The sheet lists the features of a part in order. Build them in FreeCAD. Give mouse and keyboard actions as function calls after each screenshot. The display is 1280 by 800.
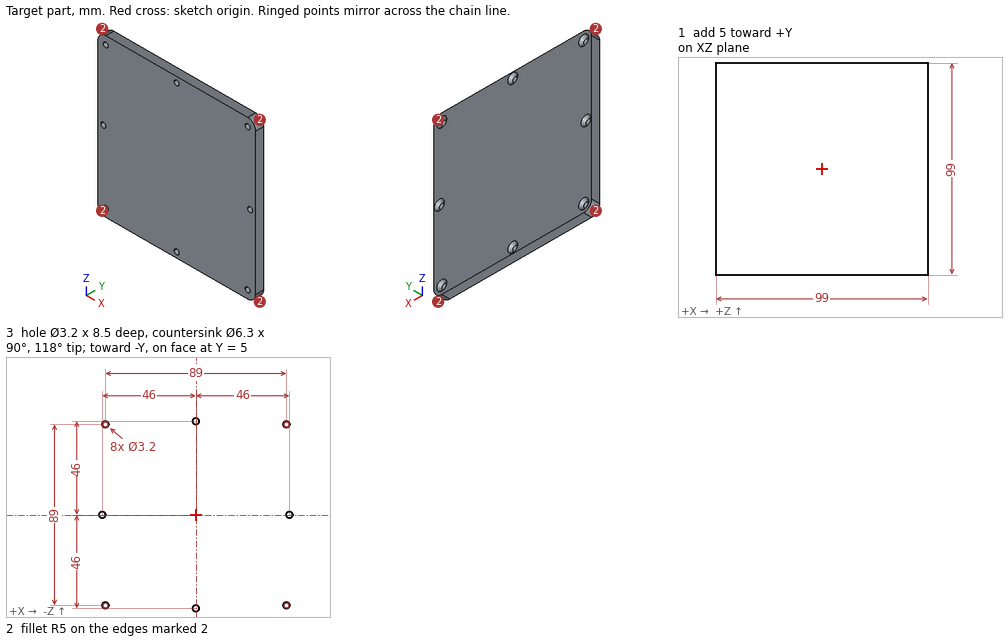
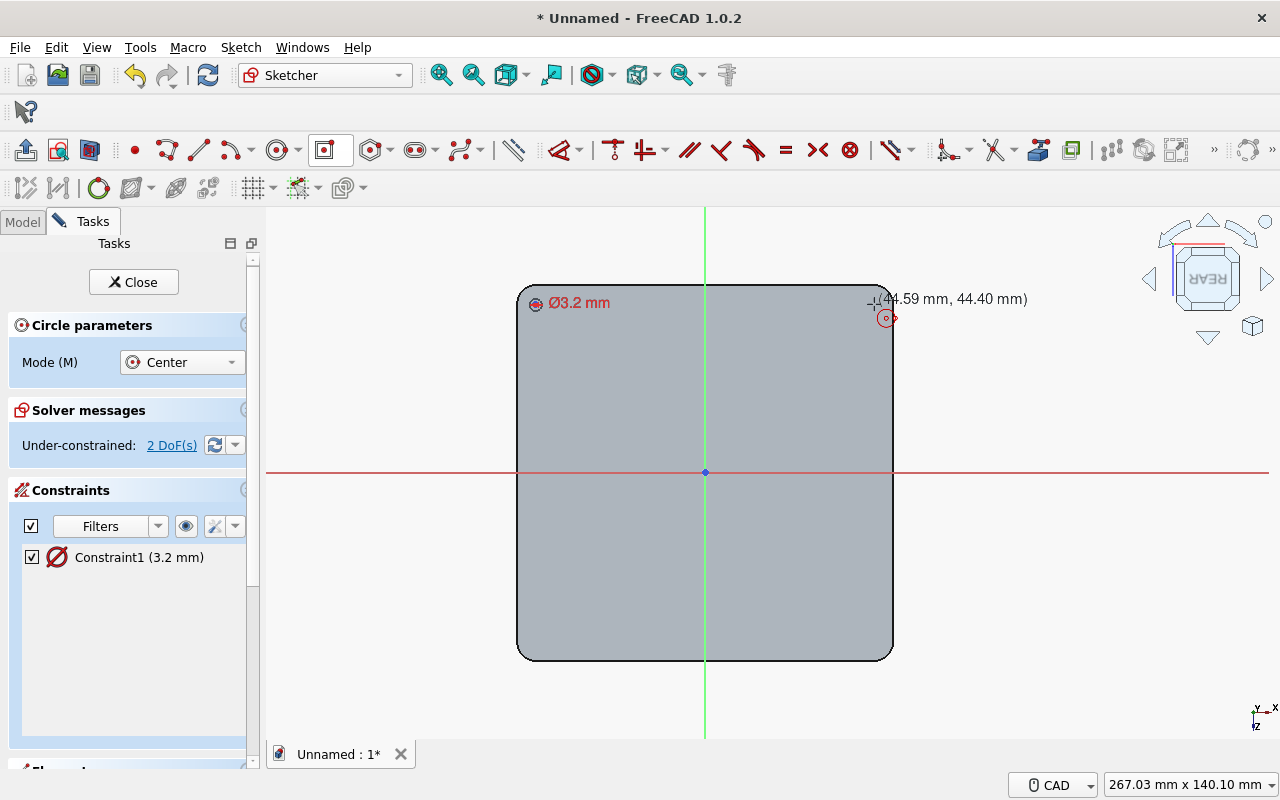
click(874, 304)
move(878, 300)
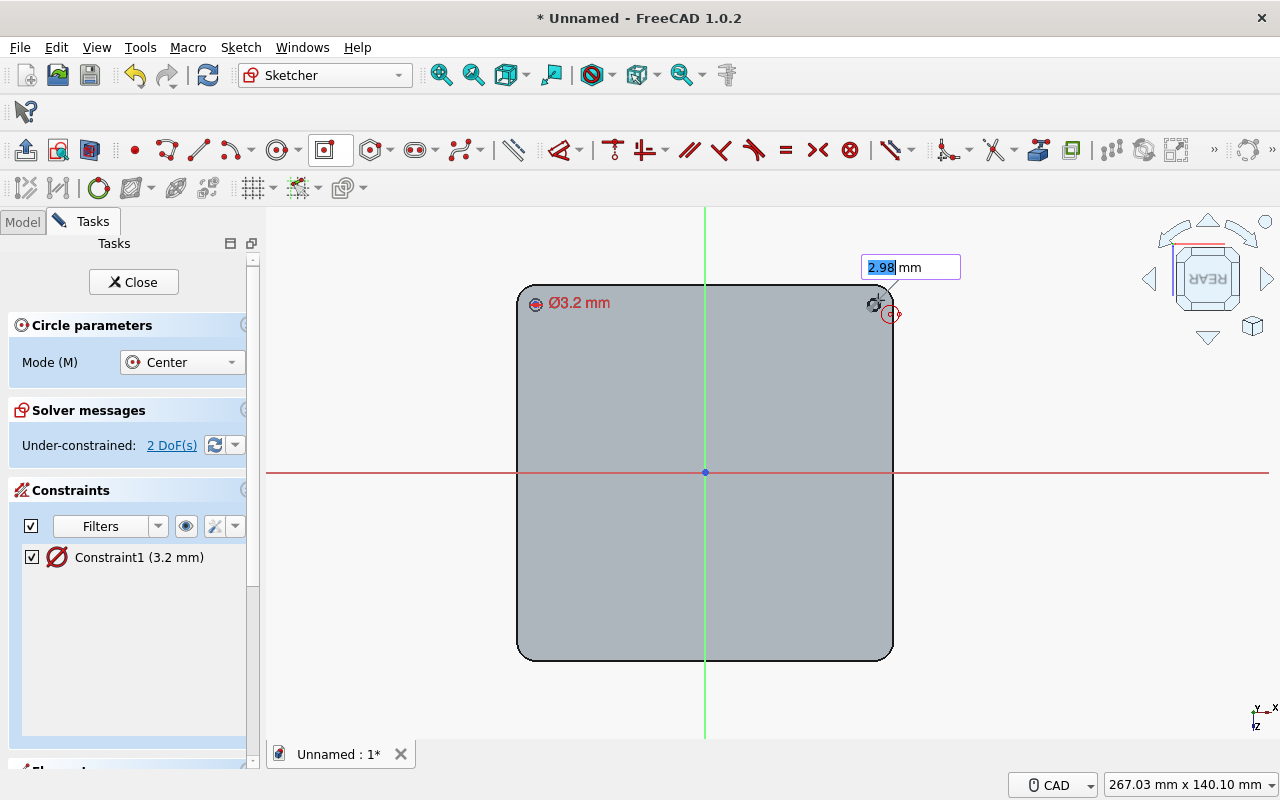
text(3.2)
key(Return)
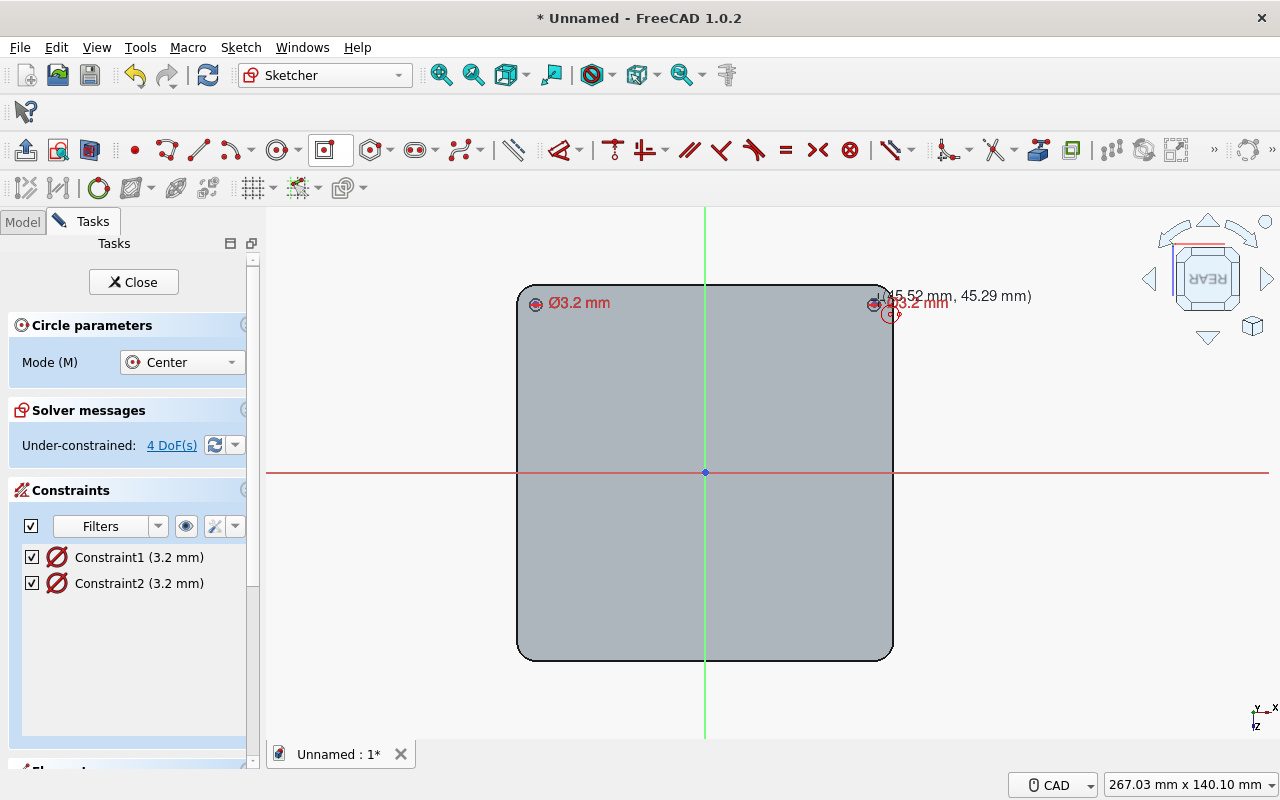
scroll(705, 298, up, 7)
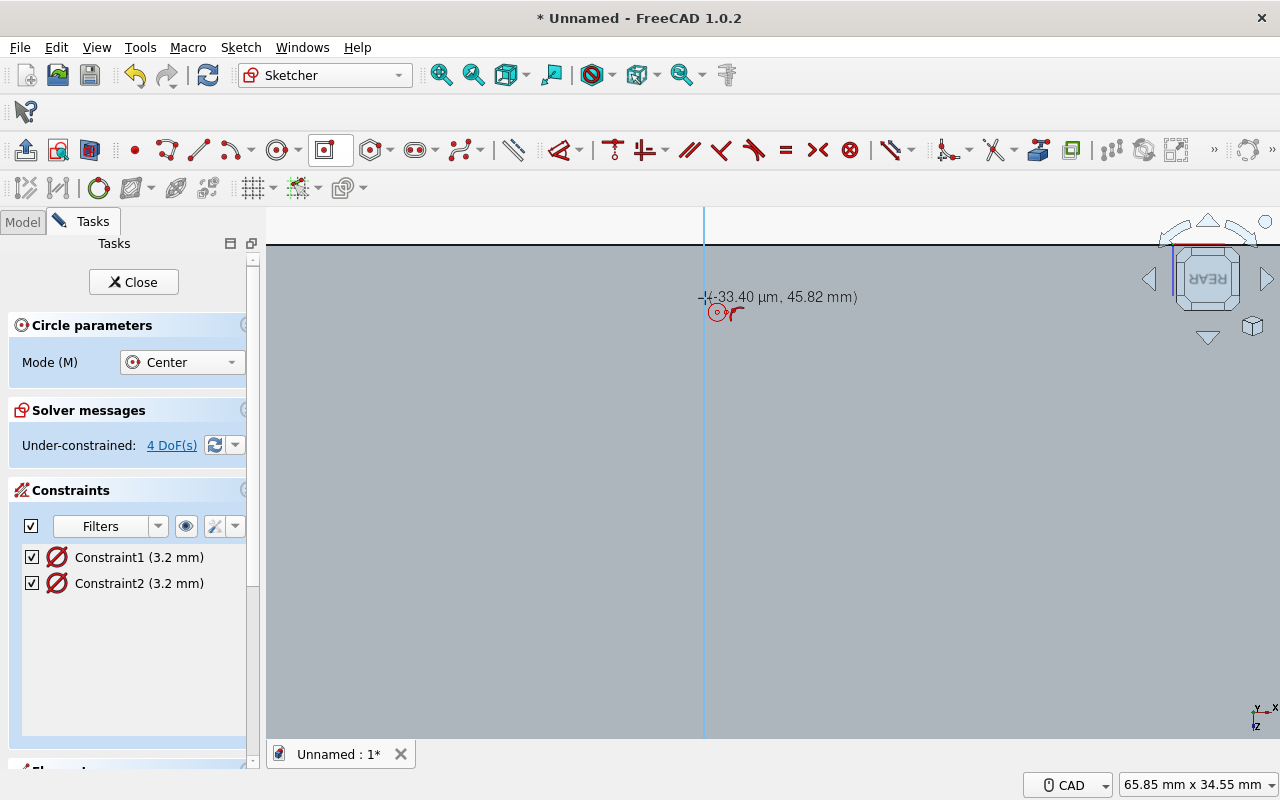
scroll(705, 298, down, 7)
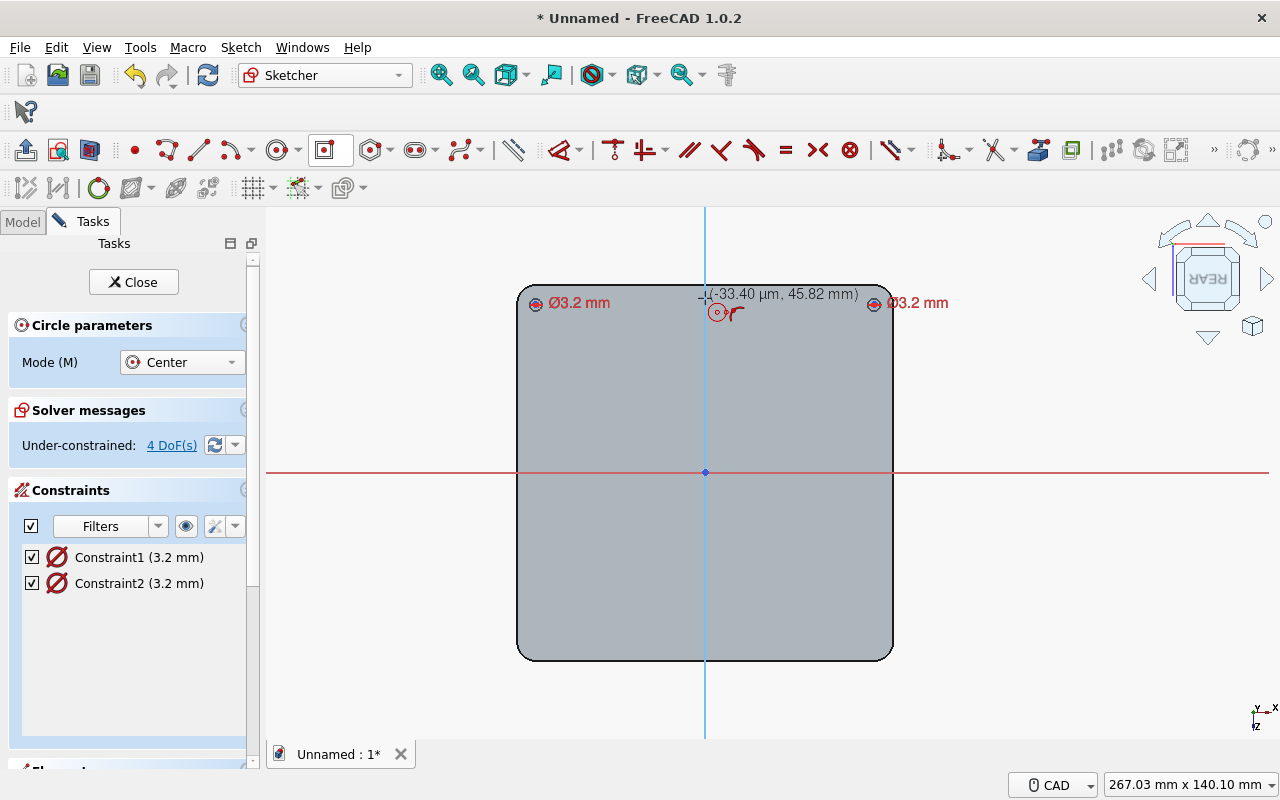
click(705, 298)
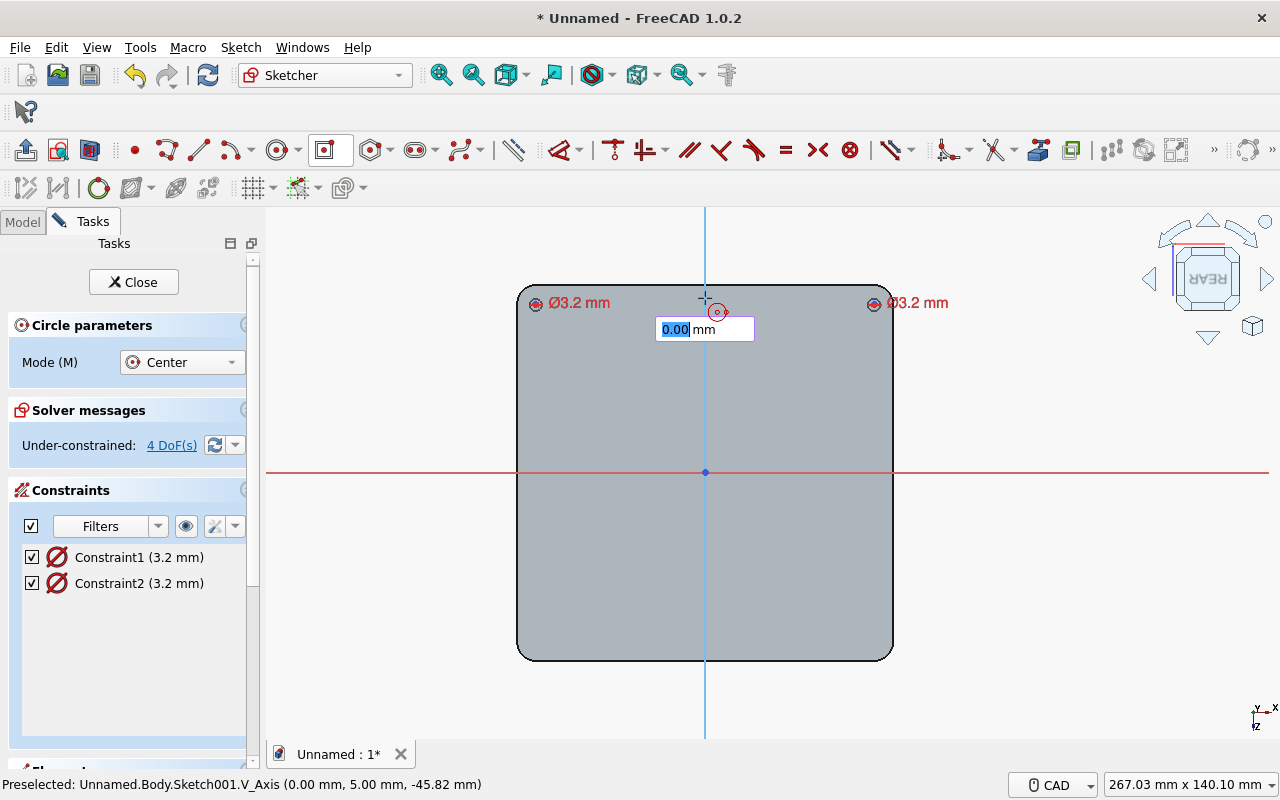
scroll(711, 296, up, 6)
move(709, 296)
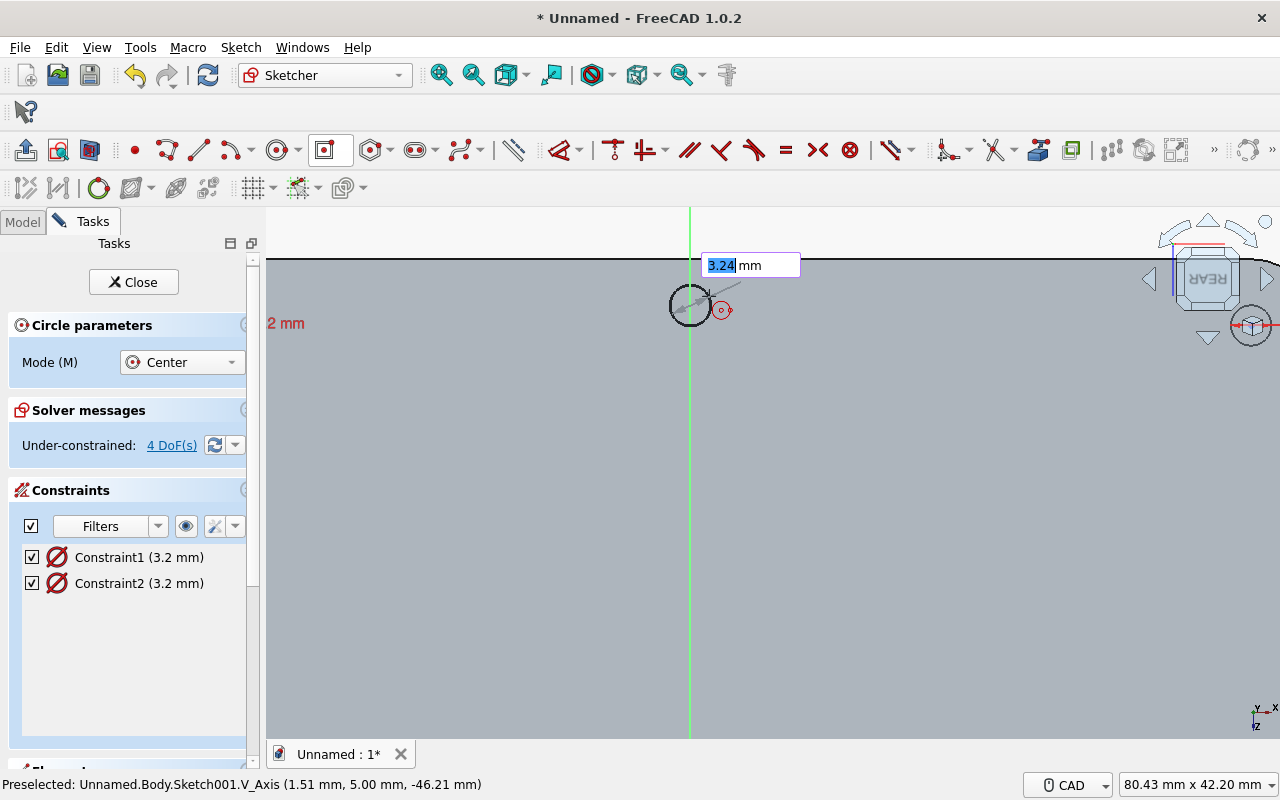
text(3.2)
key(Return)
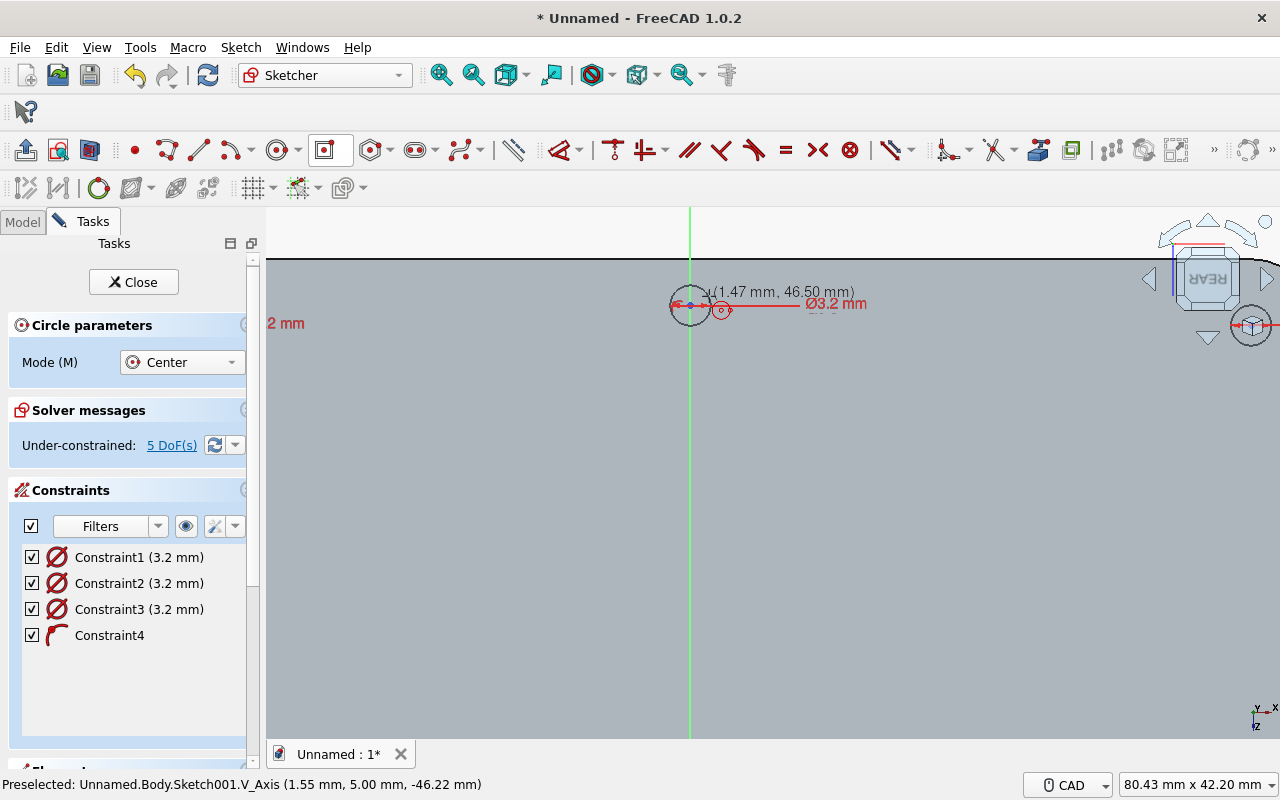
scroll(711, 296, down, 6)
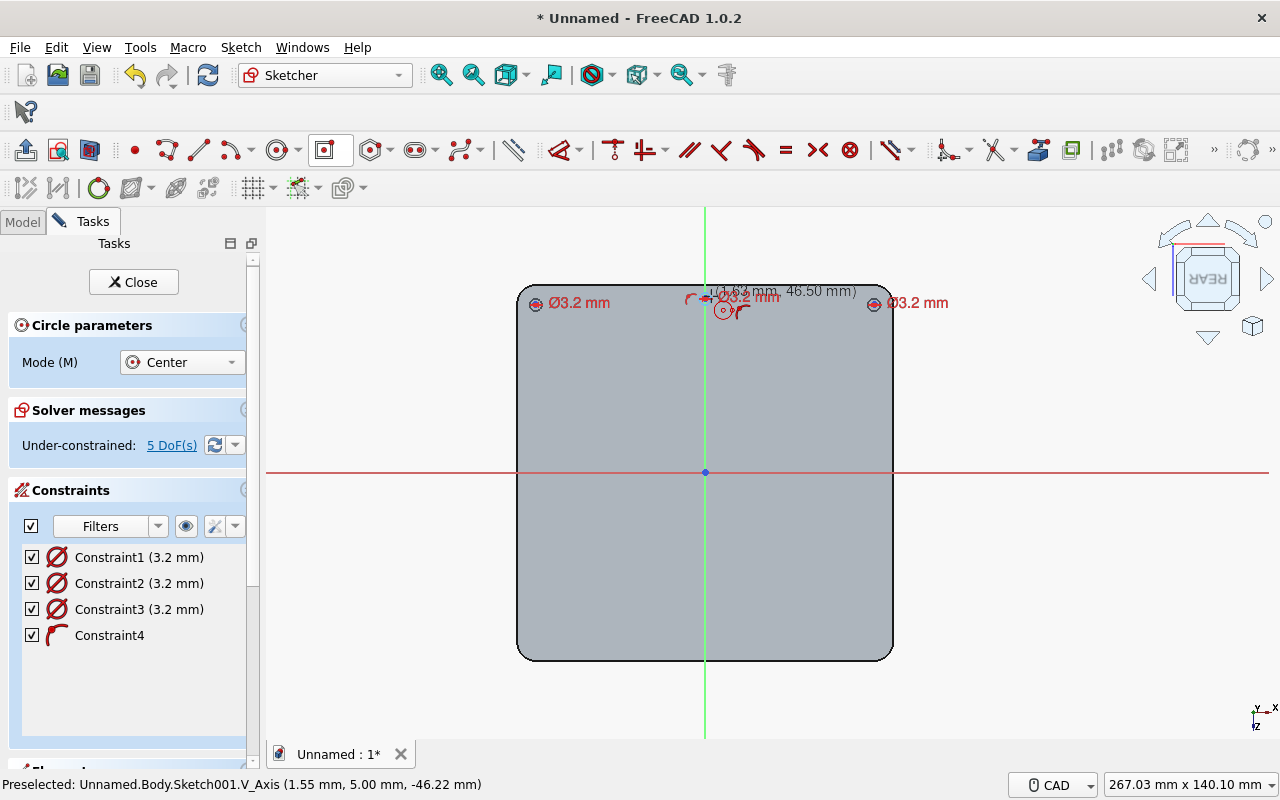
scroll(530, 473, up, 7)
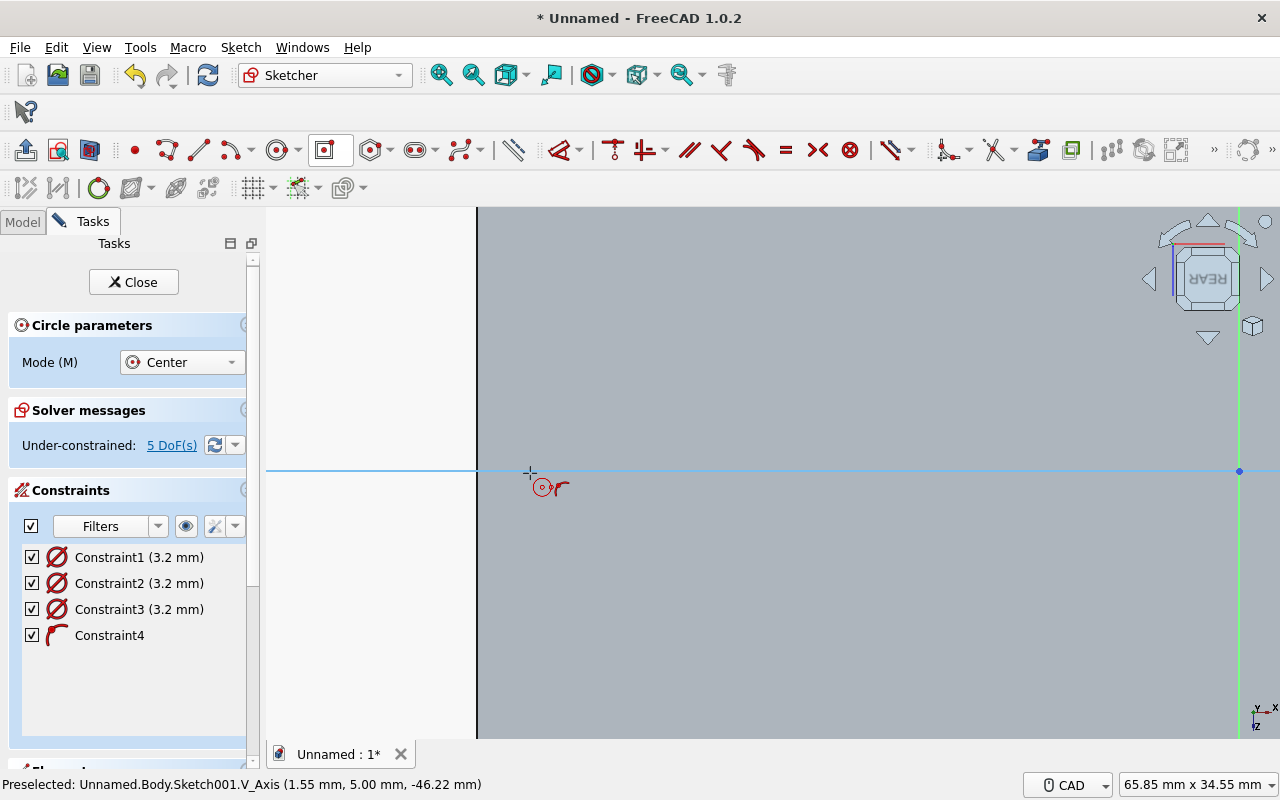
scroll(529, 474, down, 7)